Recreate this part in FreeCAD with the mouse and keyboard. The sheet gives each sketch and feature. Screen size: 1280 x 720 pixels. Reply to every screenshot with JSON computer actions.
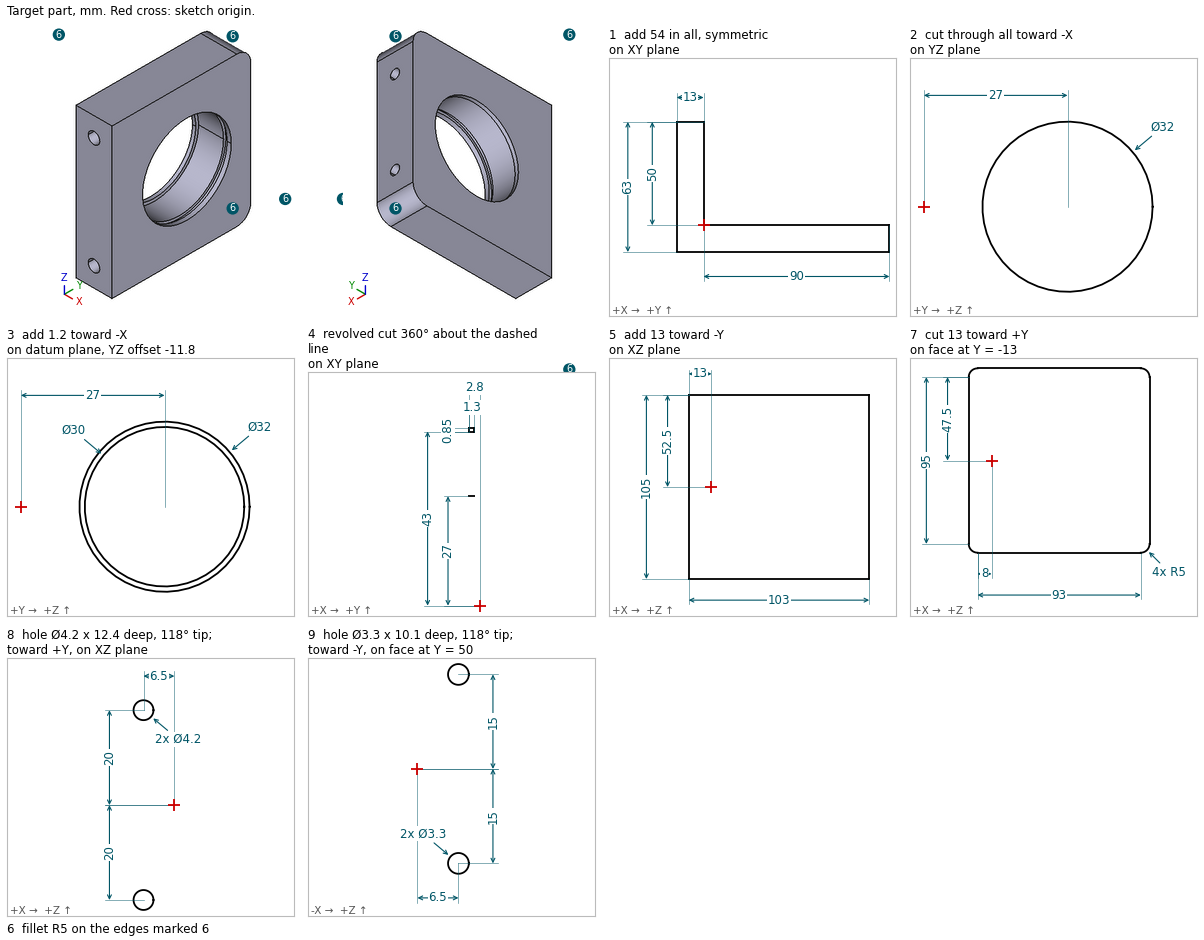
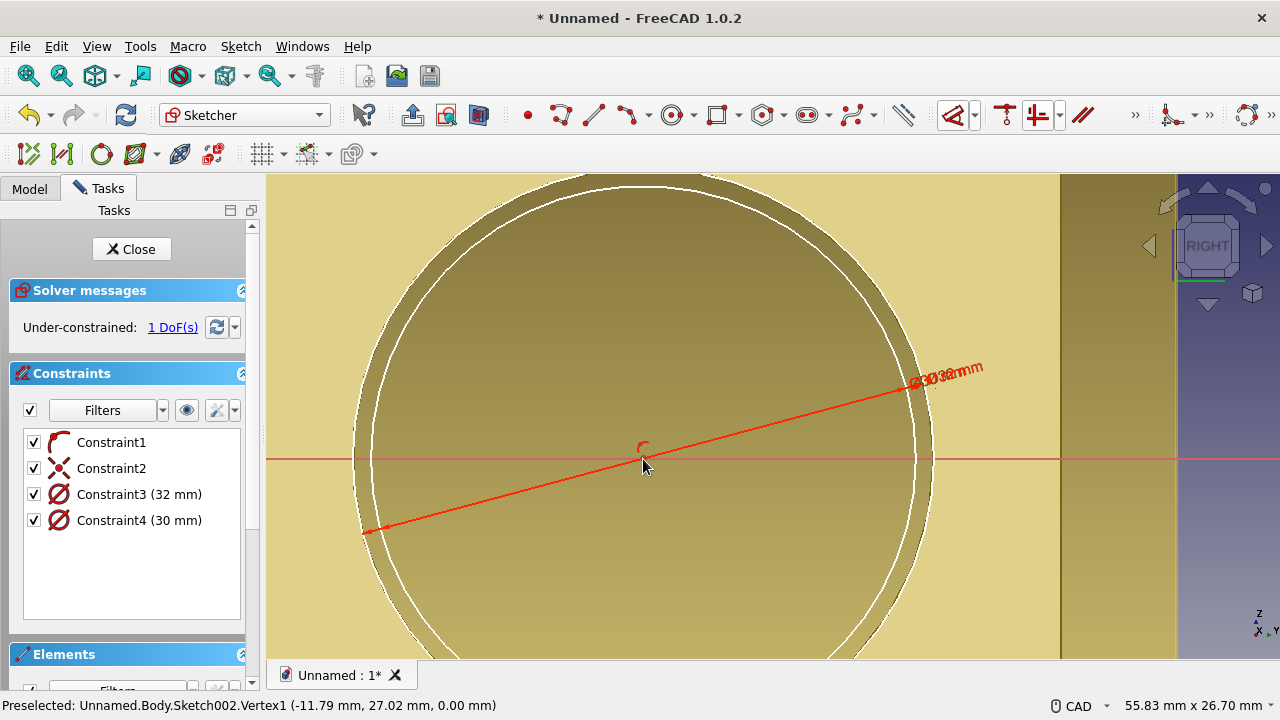
{"action": "left_click", "coordinate": [974, 116]}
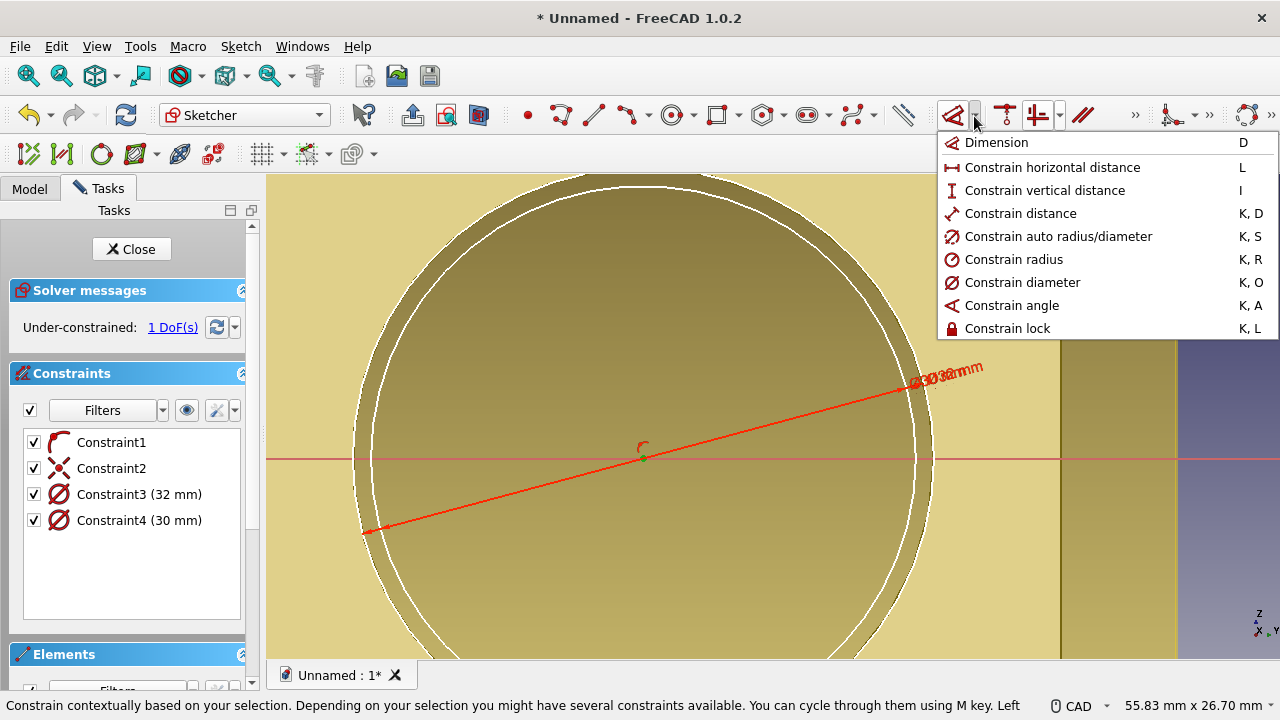
{"action": "left_click", "coordinate": [1108, 168]}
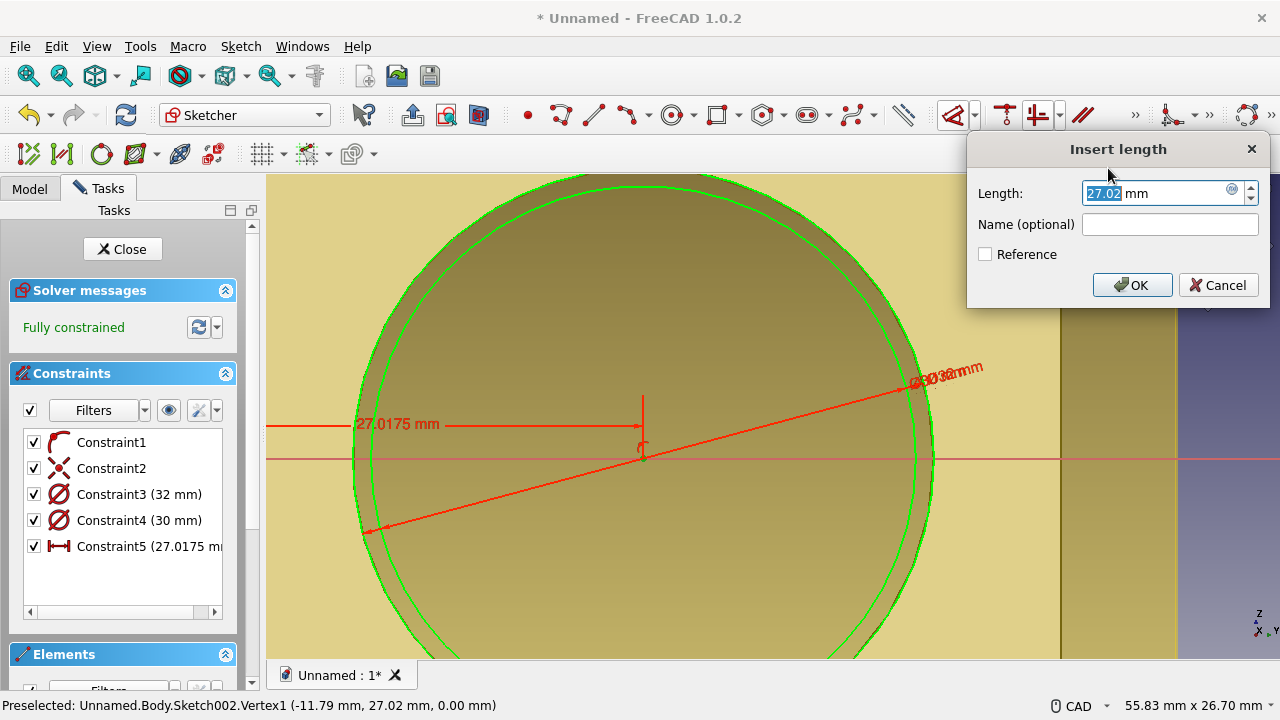
{"action": "type", "text": "27"}
{"action": "key", "text": "Return"}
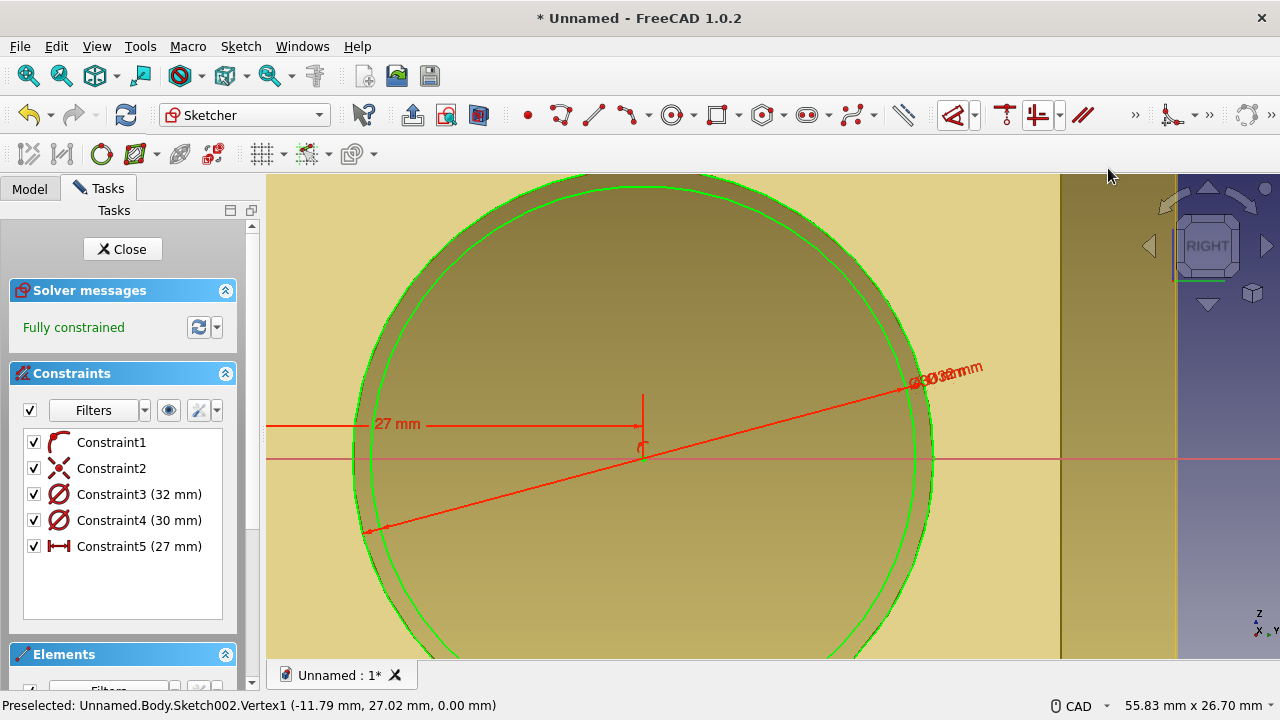
{"action": "left_click", "coordinate": [123, 249]}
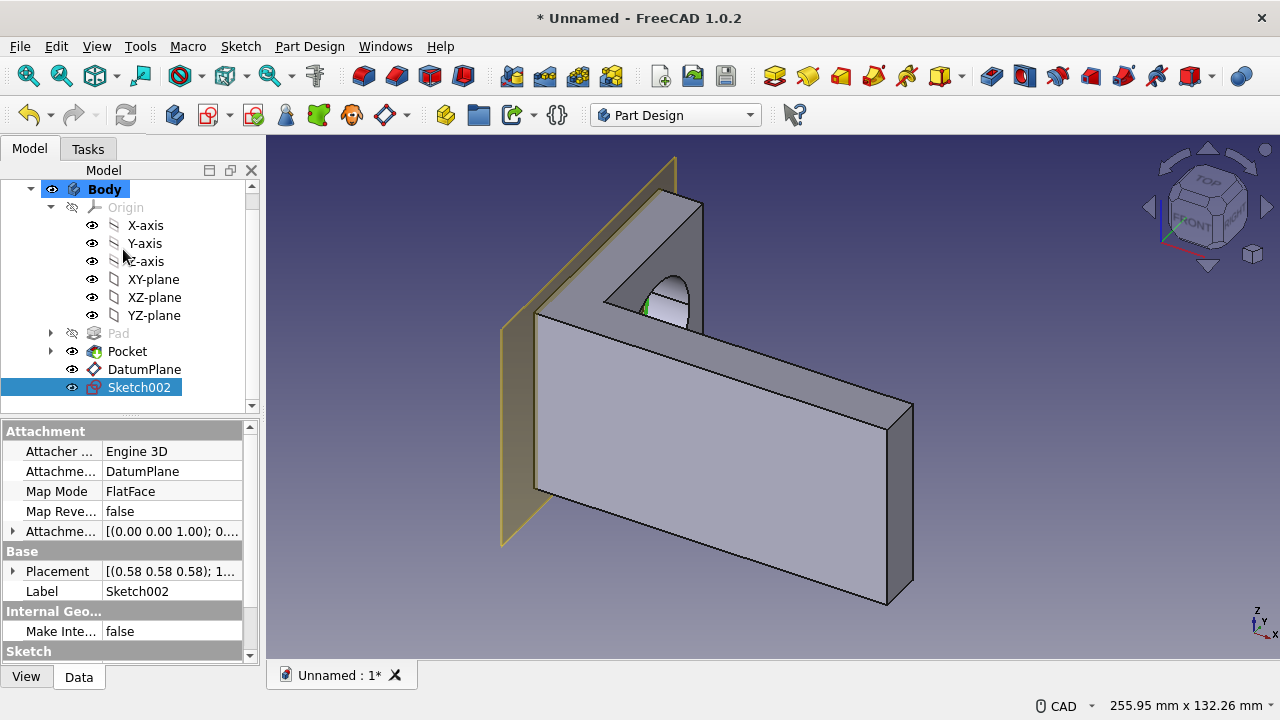
{"action": "left_click", "coordinate": [775, 76]}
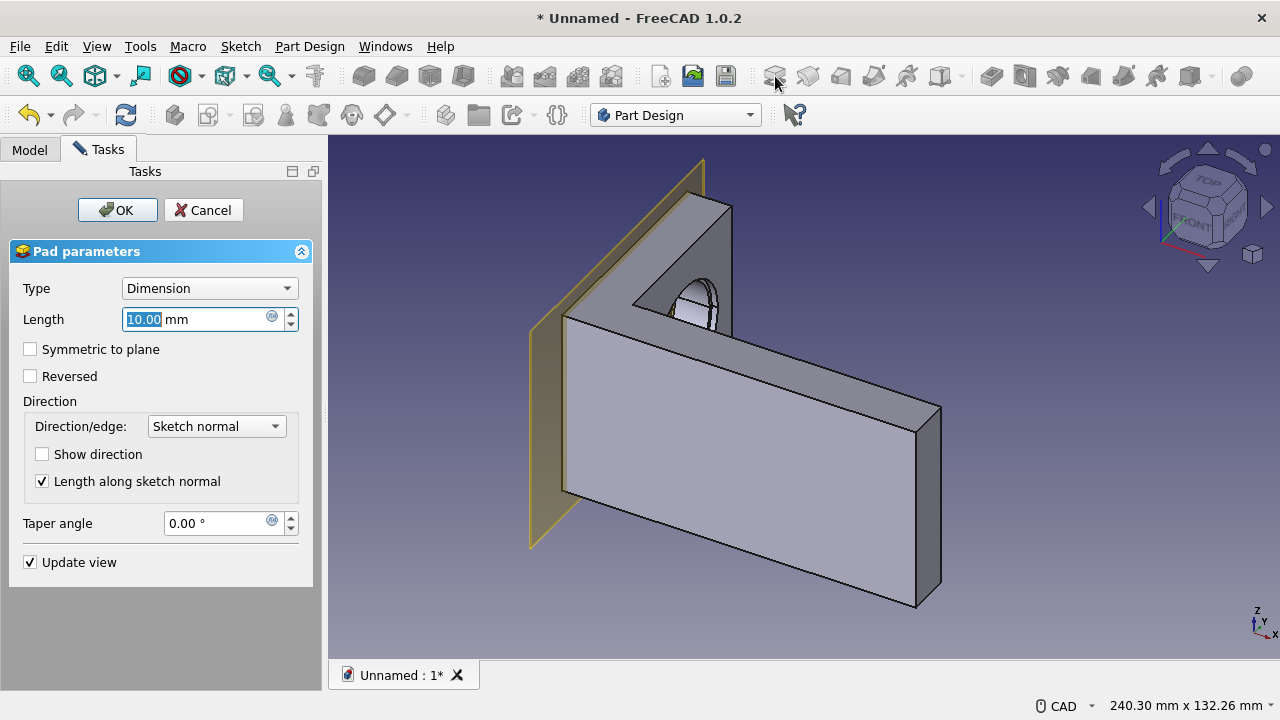
{"action": "type", "text": "1.2"}
{"action": "key", "text": "Tab"}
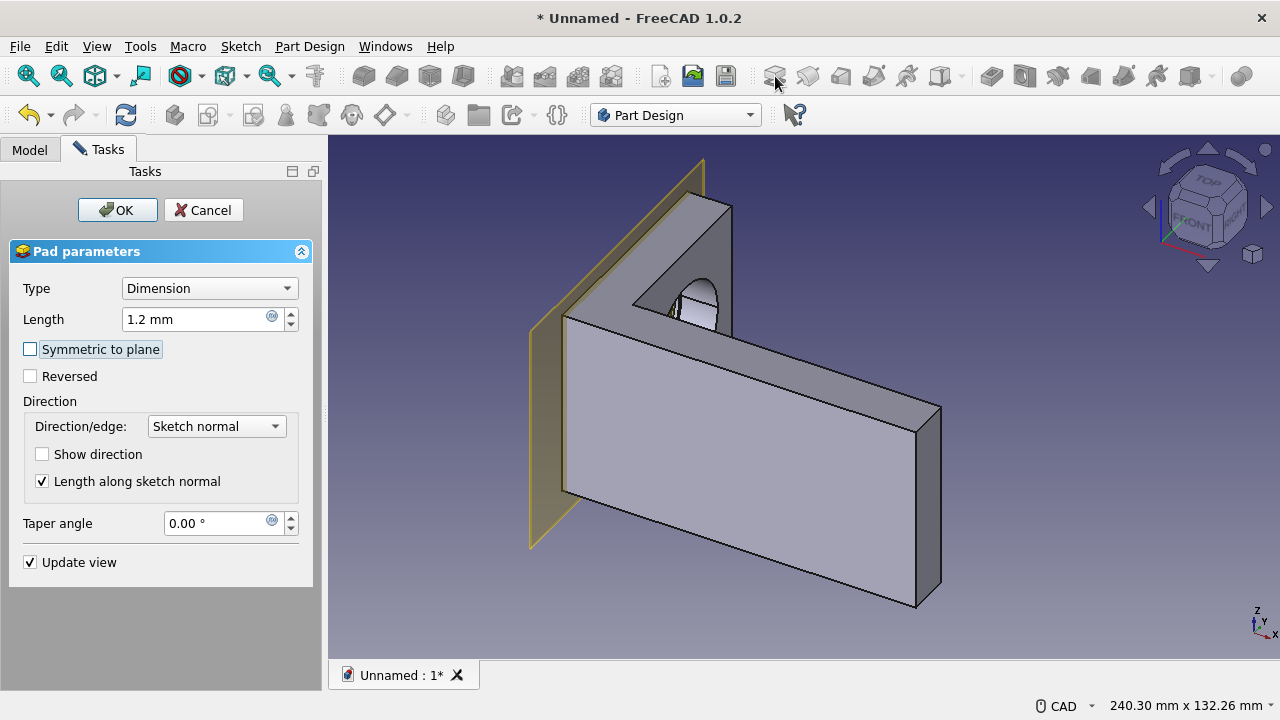
{"action": "left_click", "coordinate": [31, 376]}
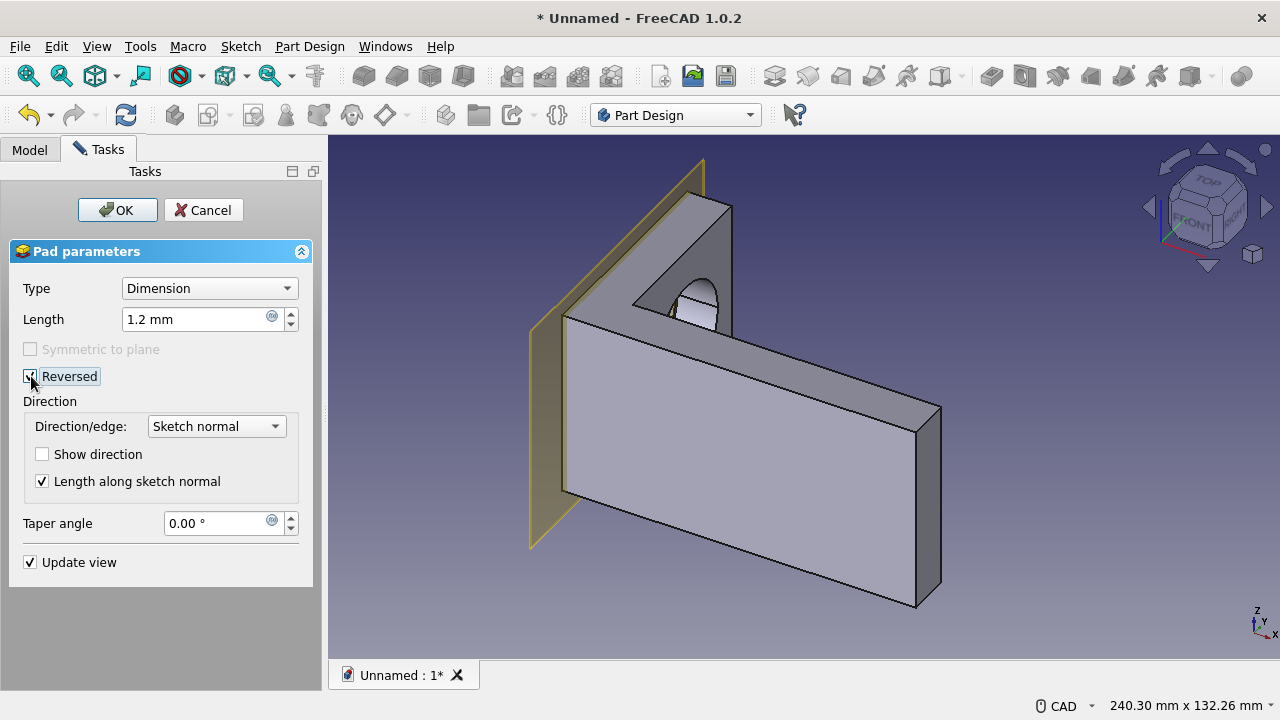
{"action": "left_click", "coordinate": [118, 210]}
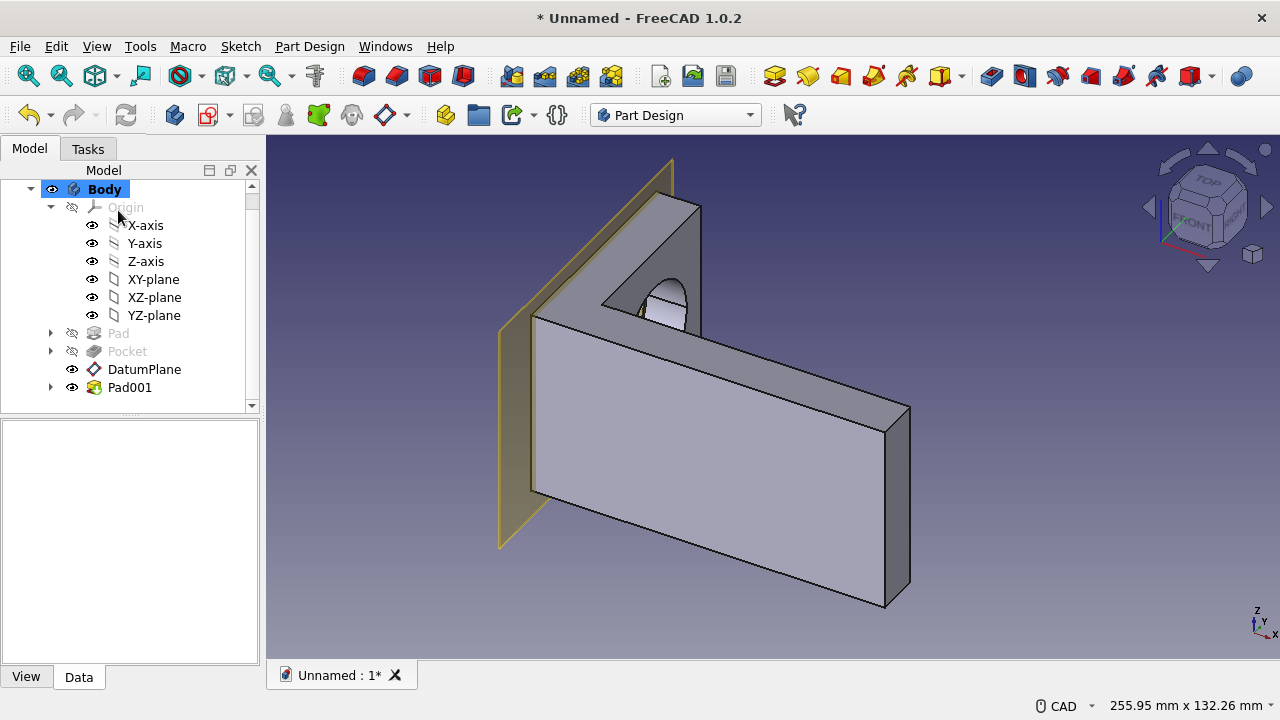
{"action": "left_click", "coordinate": [117, 369]}
{"action": "key", "text": "space"}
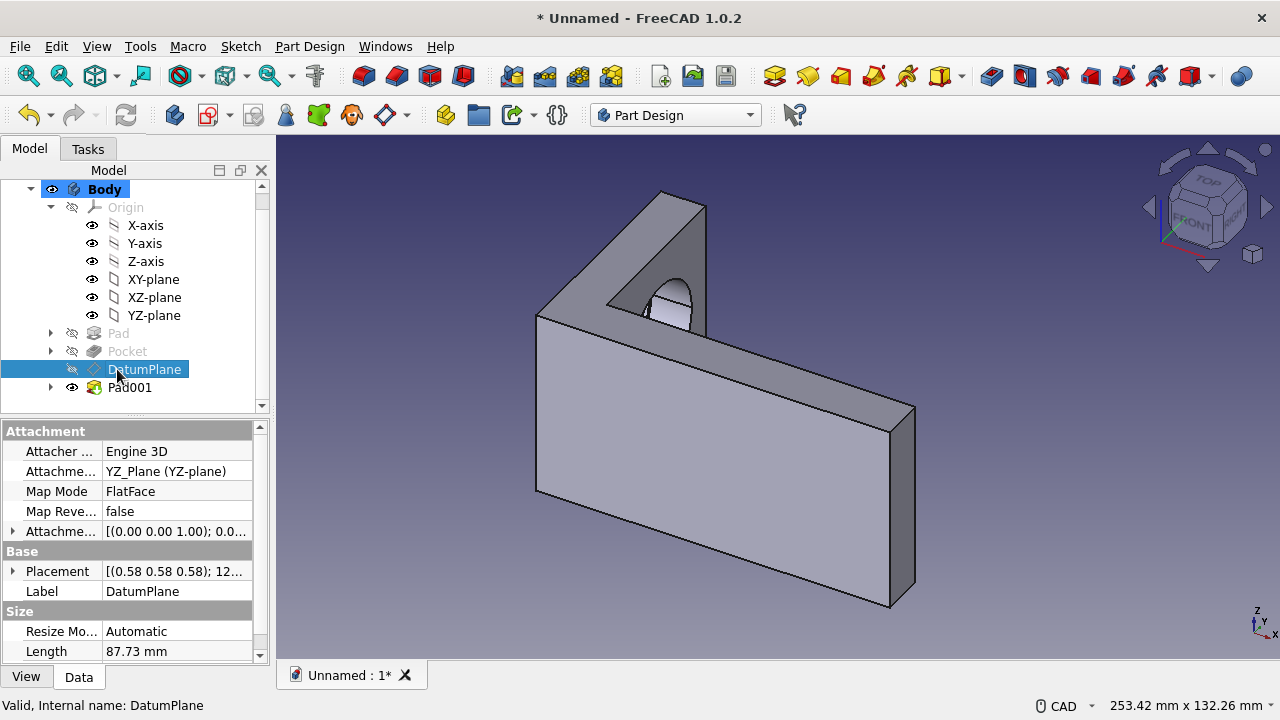
{"action": "left_click", "coordinate": [316, 619]}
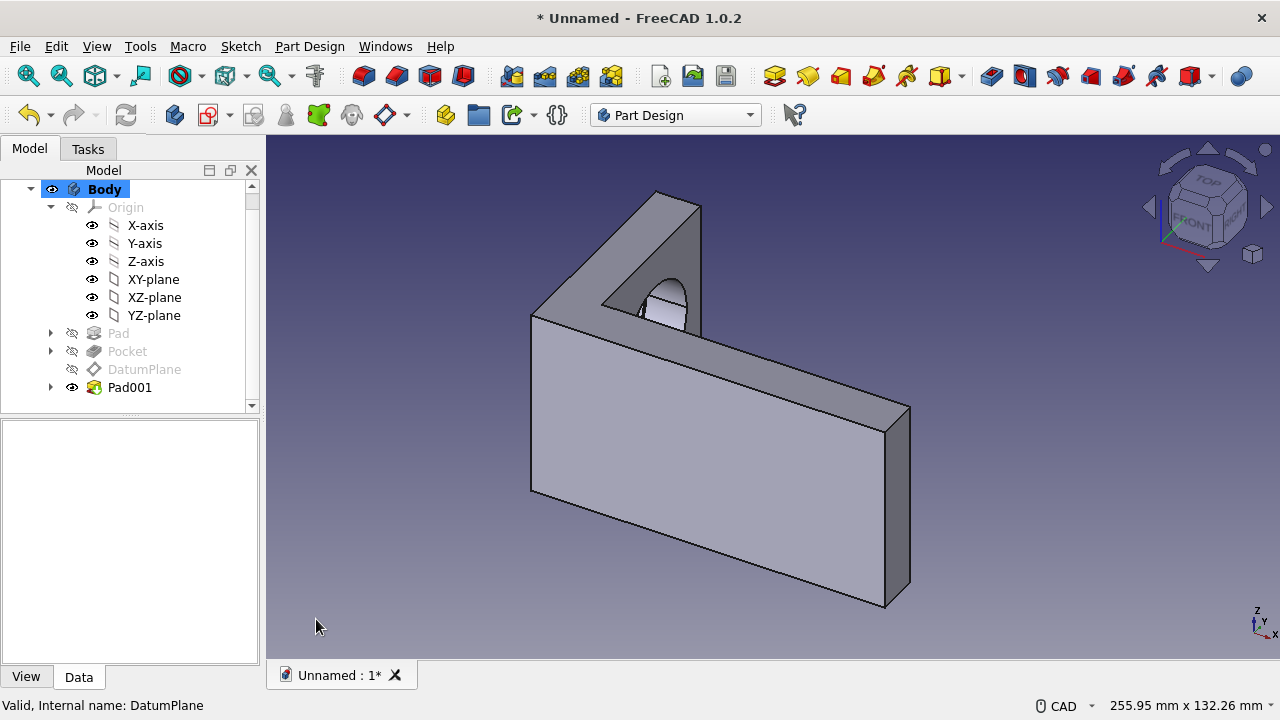
{"action": "left_click", "coordinate": [208, 116]}